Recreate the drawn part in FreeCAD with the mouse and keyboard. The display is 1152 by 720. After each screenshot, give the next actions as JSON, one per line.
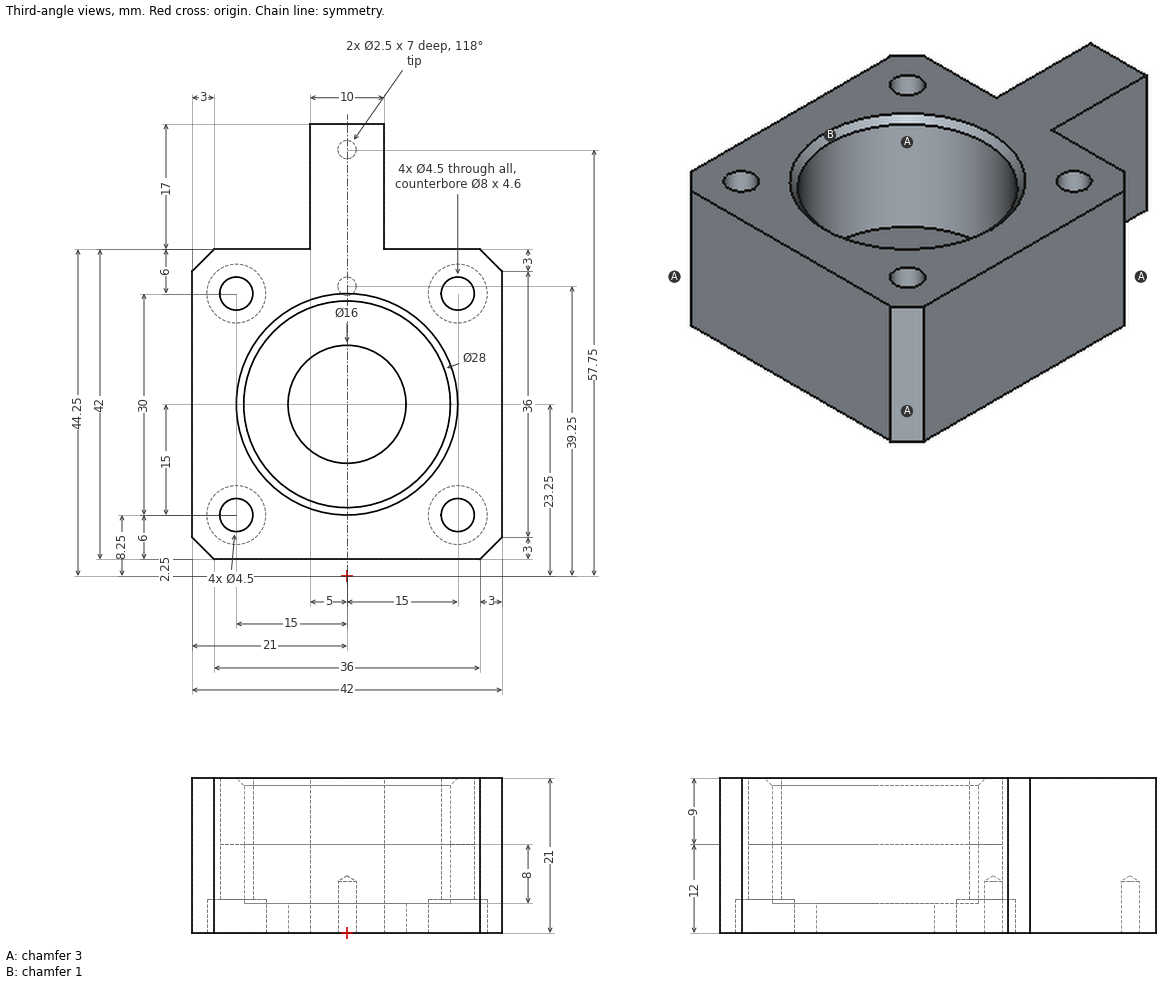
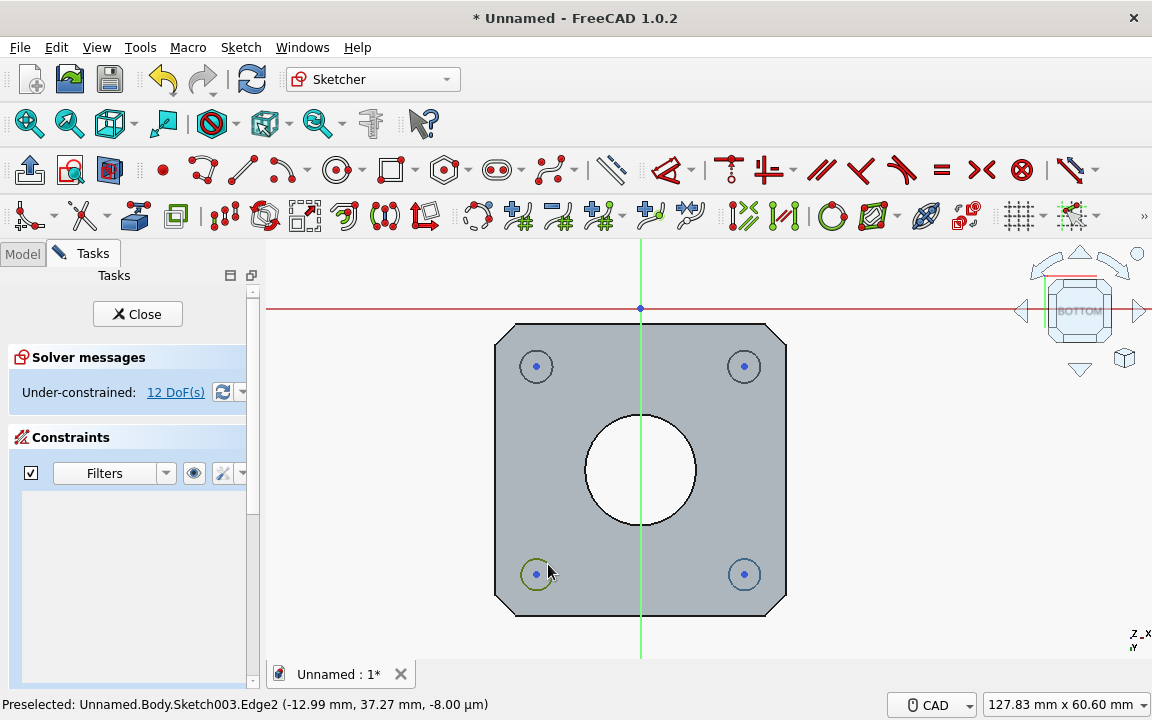
{"action": "left_click", "coordinate": [548, 355]}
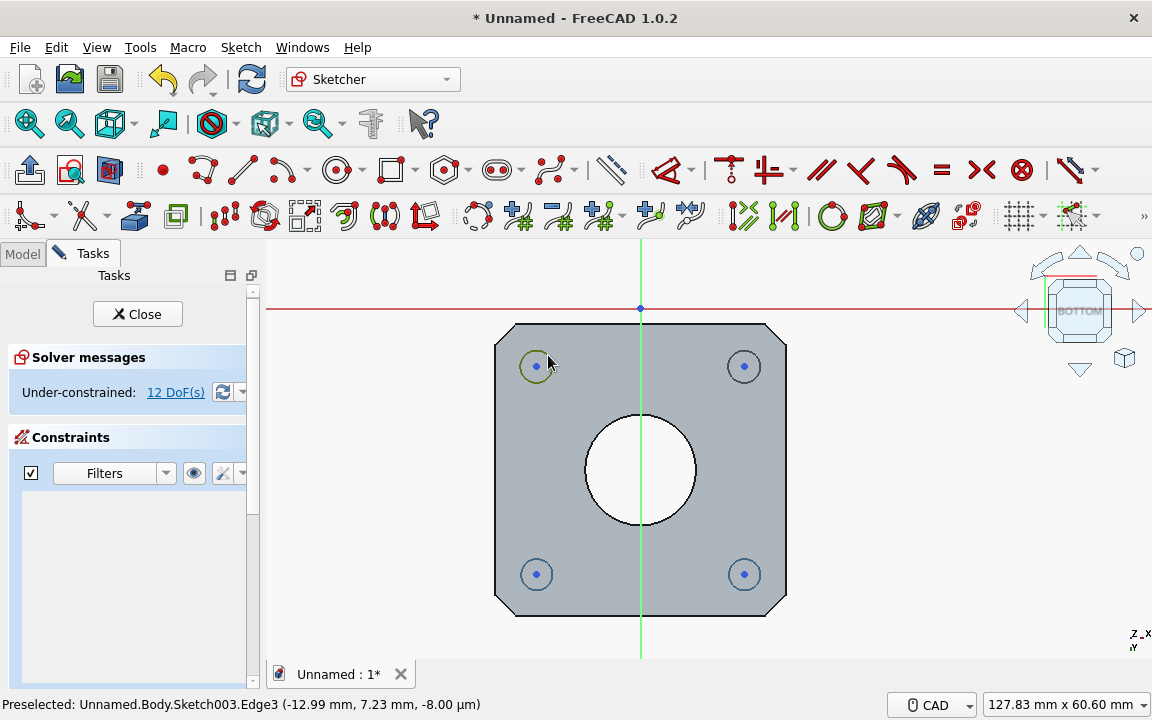
{"action": "left_click", "coordinate": [756, 355]}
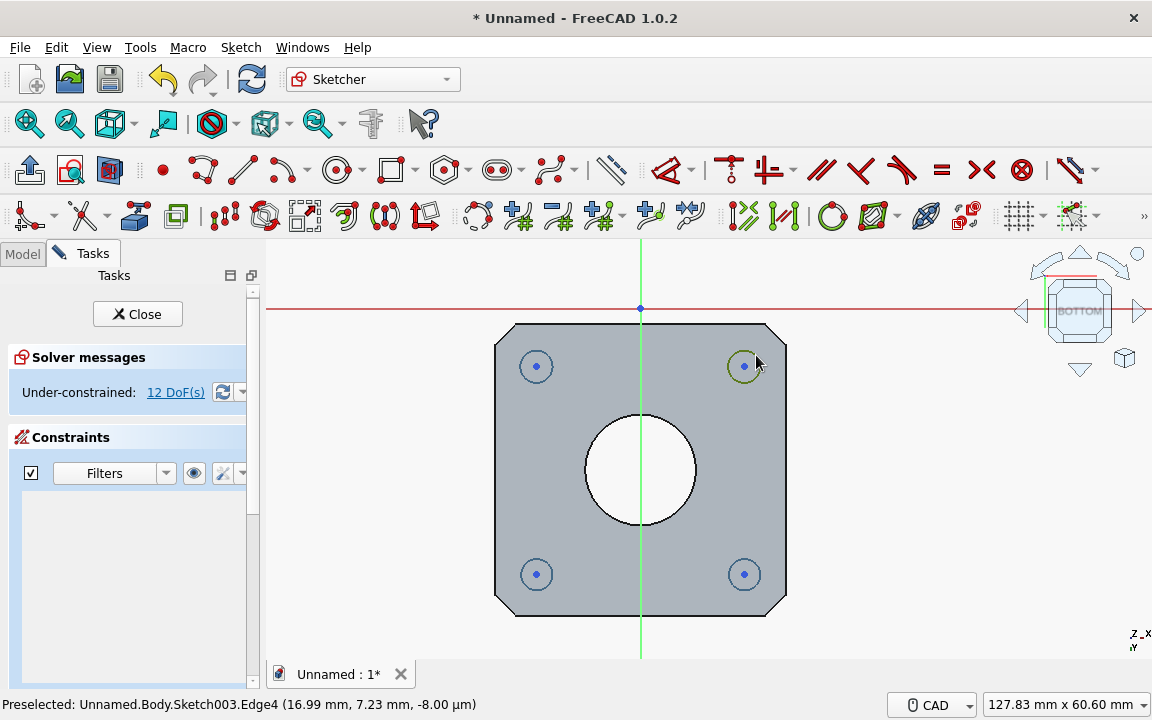
{"action": "left_click", "coordinate": [942, 170]}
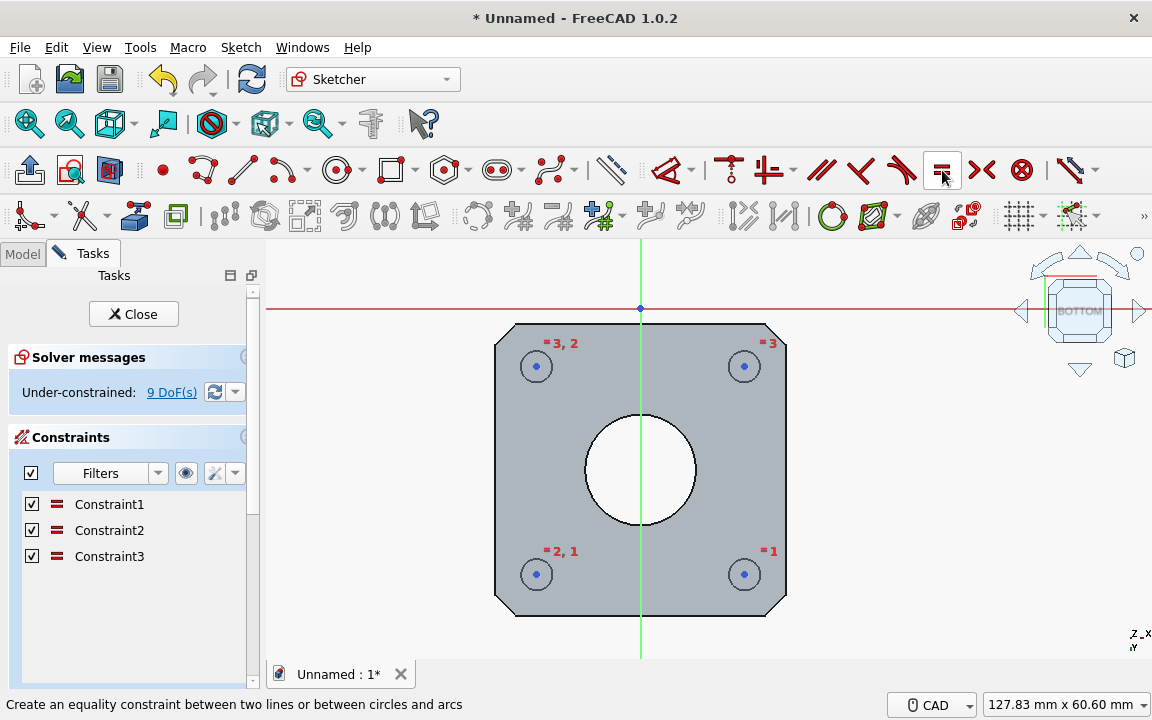
{"action": "left_click", "coordinate": [745, 575]}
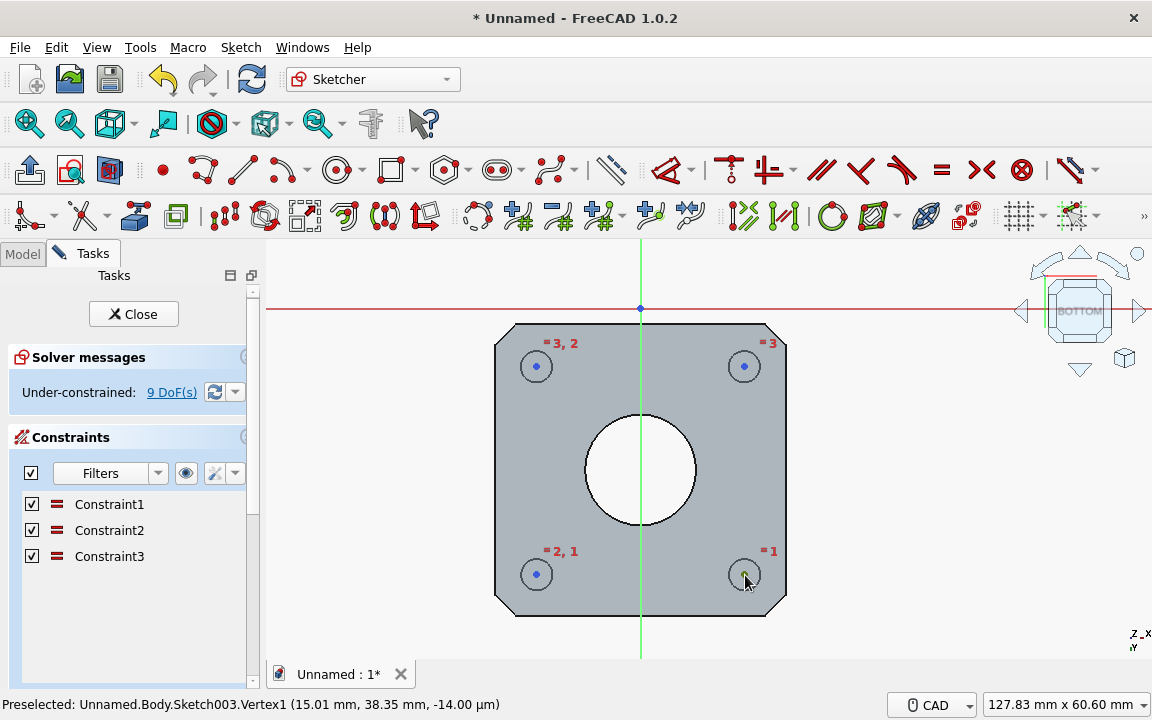
{"action": "left_click", "coordinate": [537, 575]}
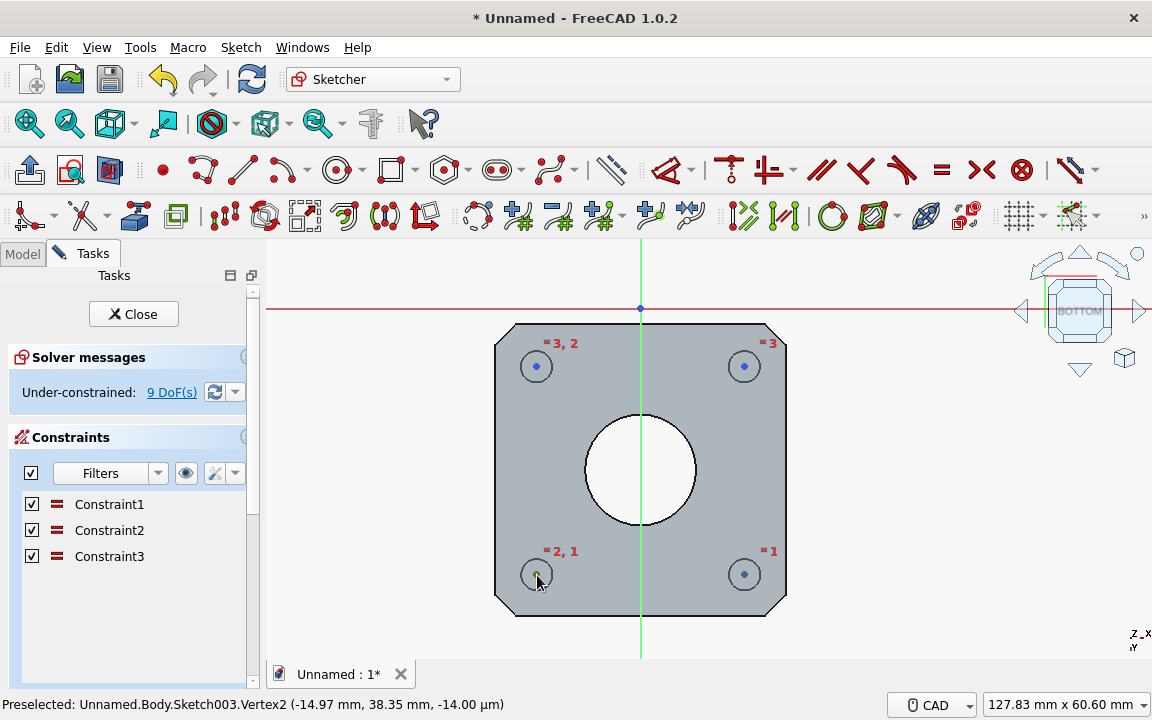
{"action": "key", "text": "h"}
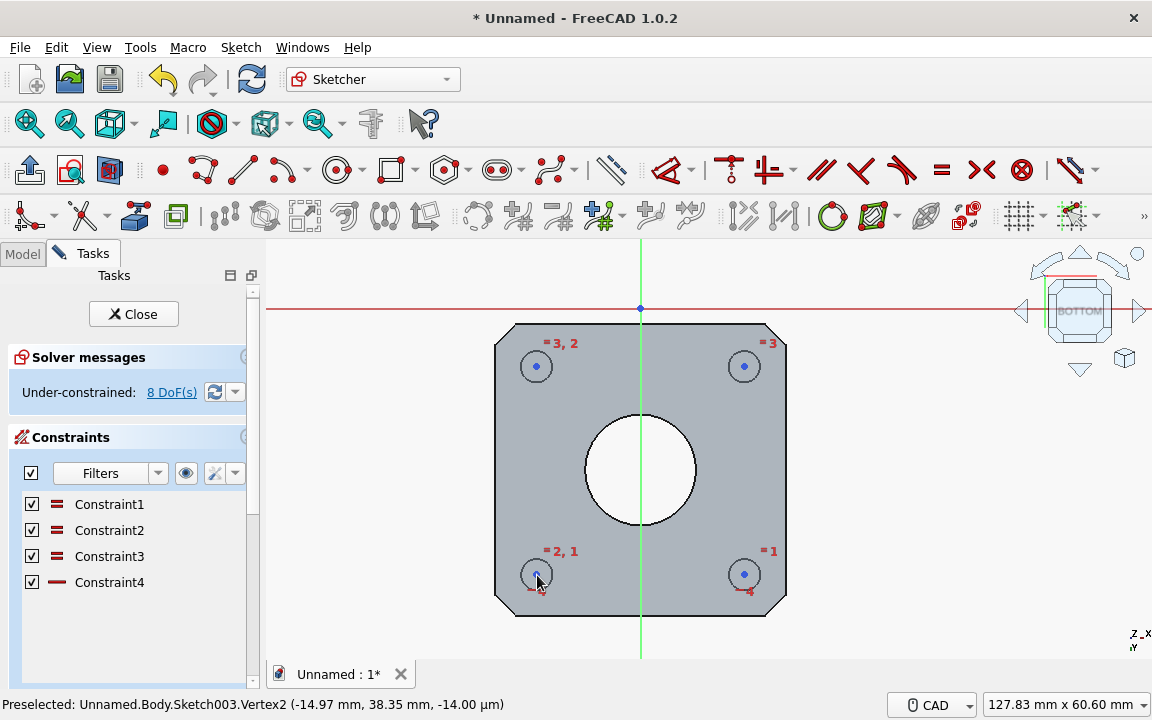
{"action": "left_click", "coordinate": [537, 575]}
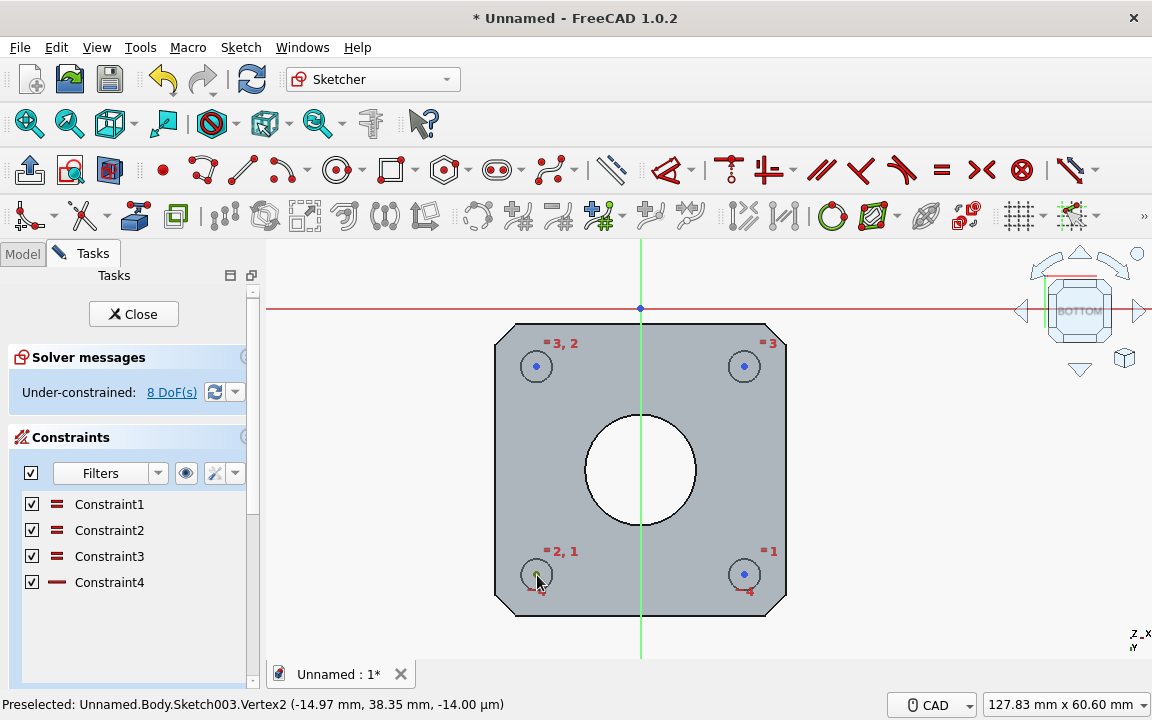
{"action": "left_click", "coordinate": [536, 367]}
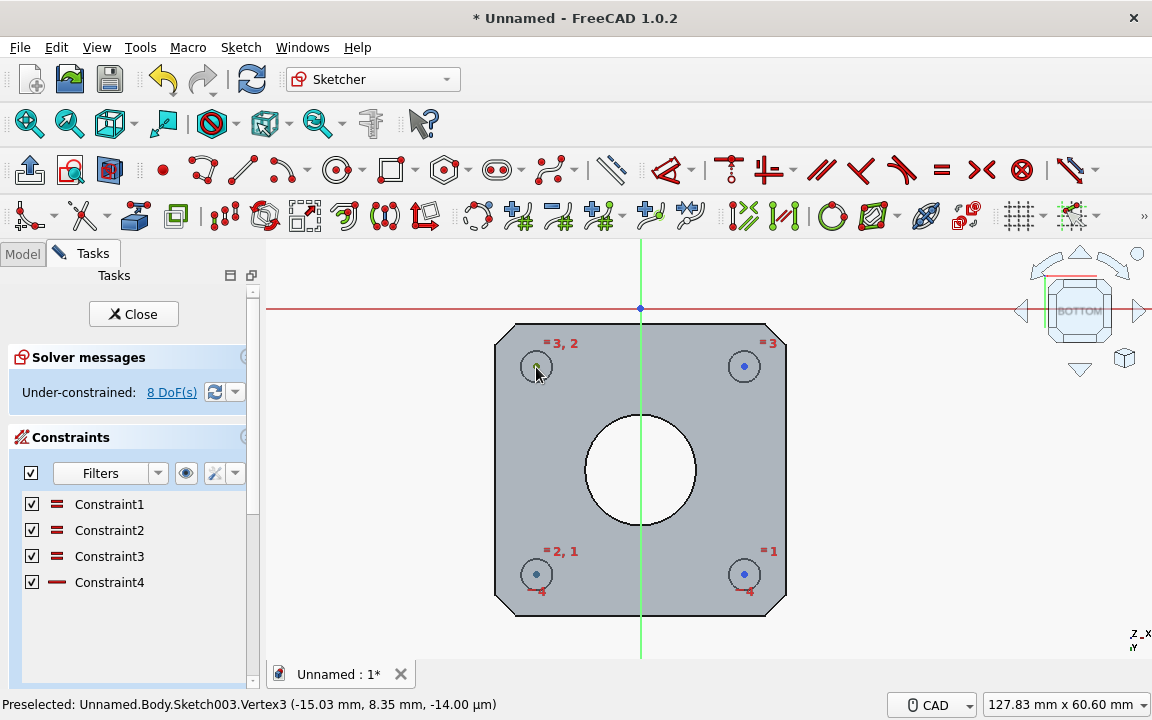
{"action": "key", "text": "v"}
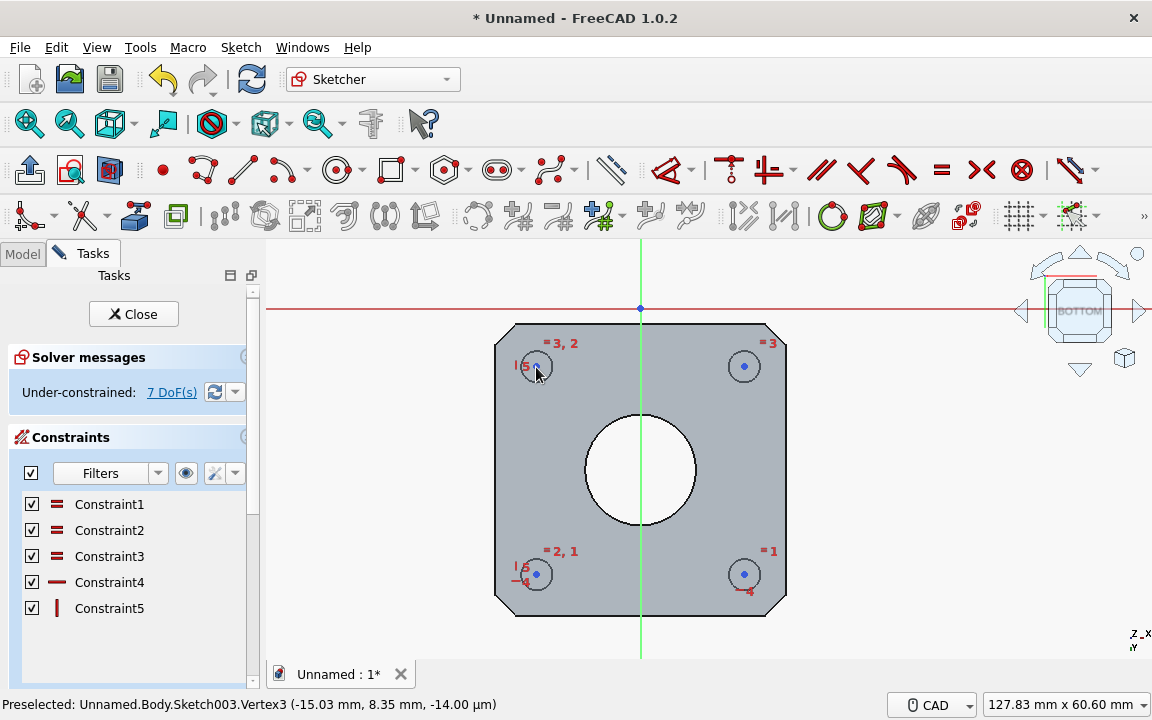
{"action": "left_click", "coordinate": [745, 575]}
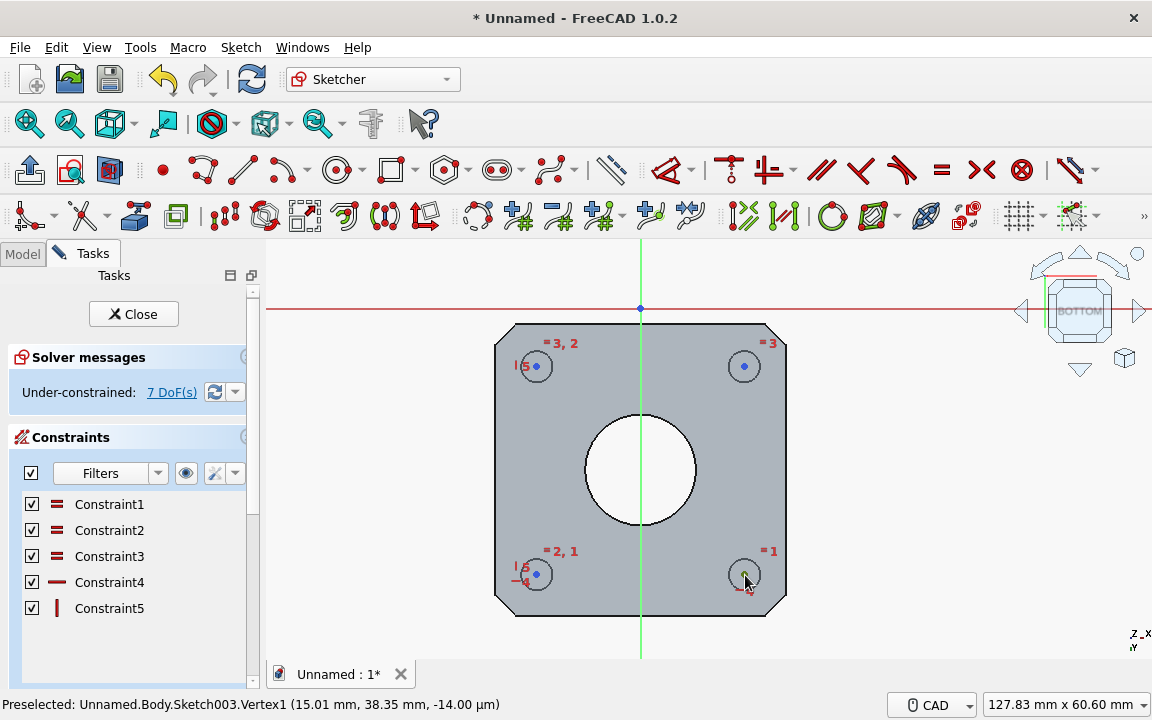
{"action": "left_click", "coordinate": [744, 367]}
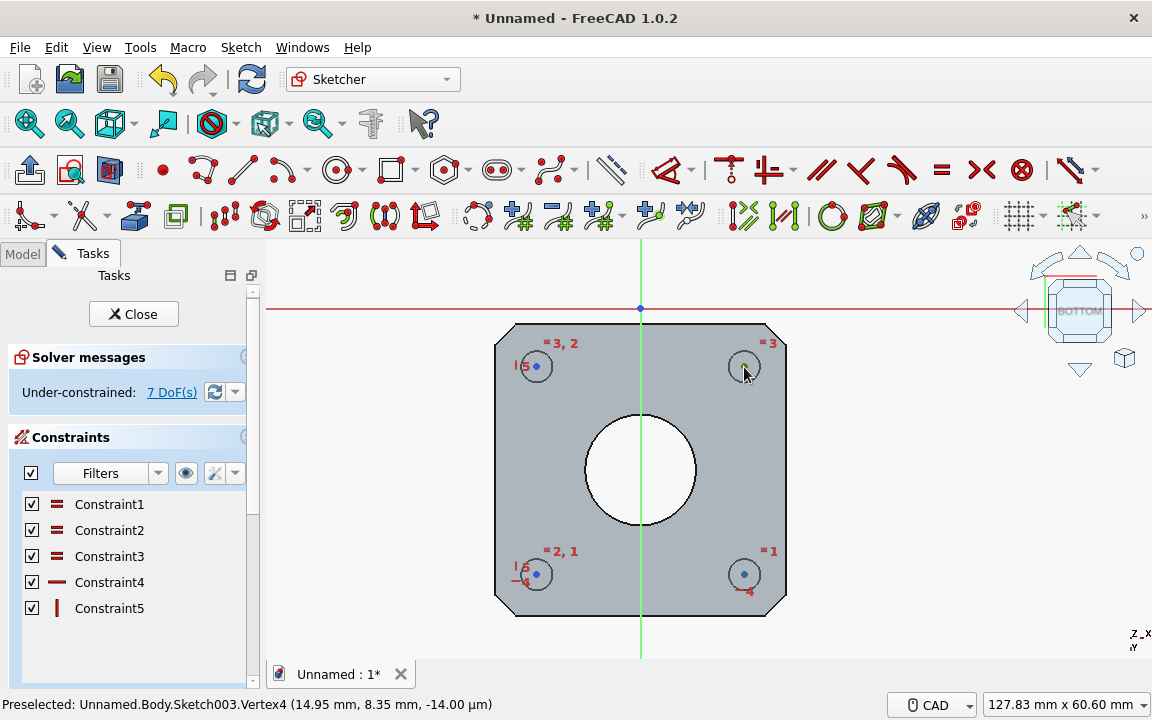
{"action": "left_click", "coordinate": [796, 170]}